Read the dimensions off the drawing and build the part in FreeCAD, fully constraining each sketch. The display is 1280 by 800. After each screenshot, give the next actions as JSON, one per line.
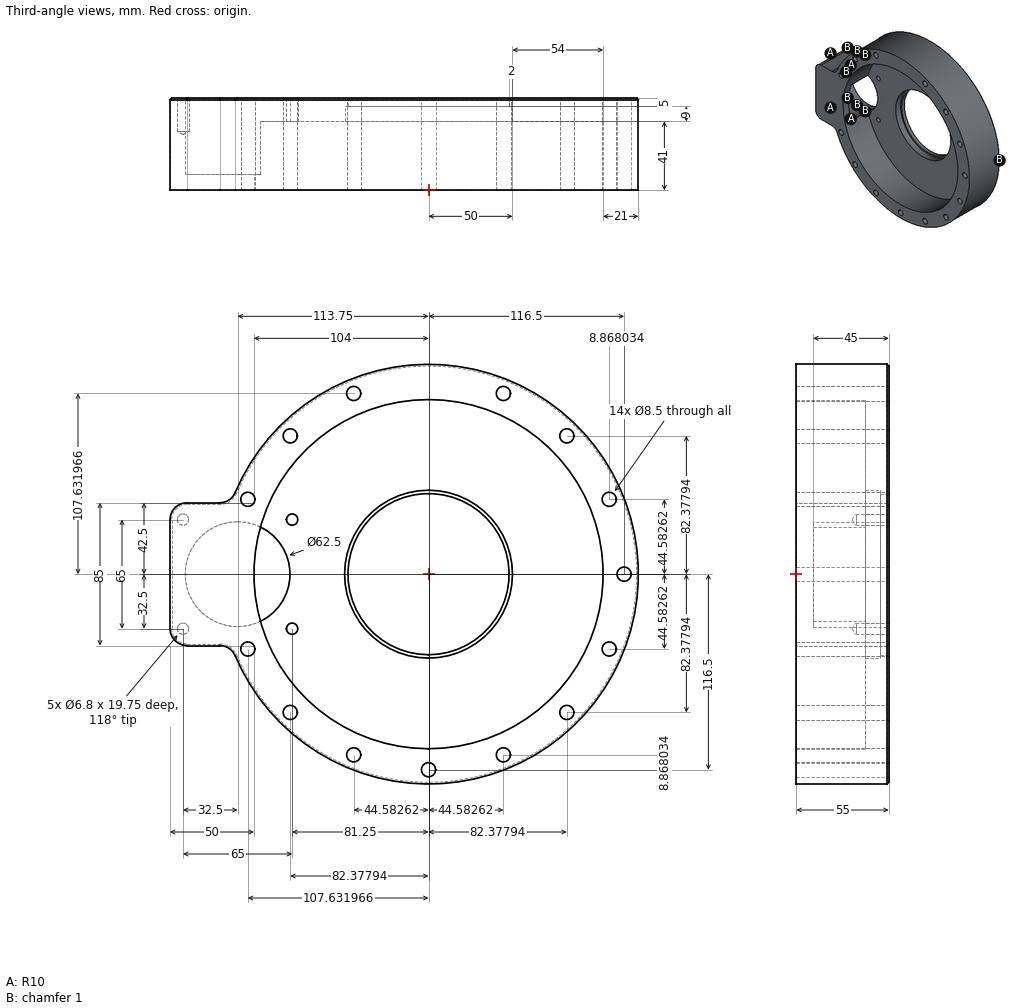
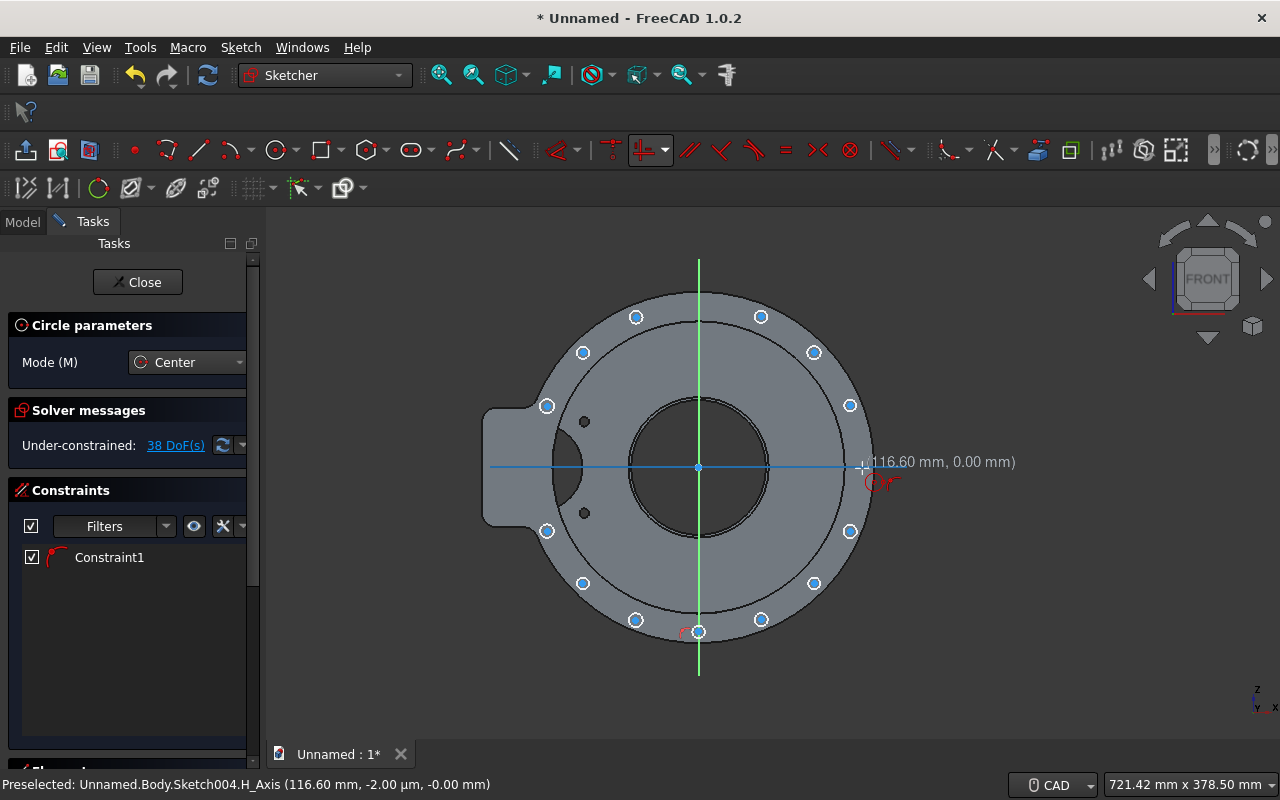
{"action": "left_click", "coordinate": [862, 467]}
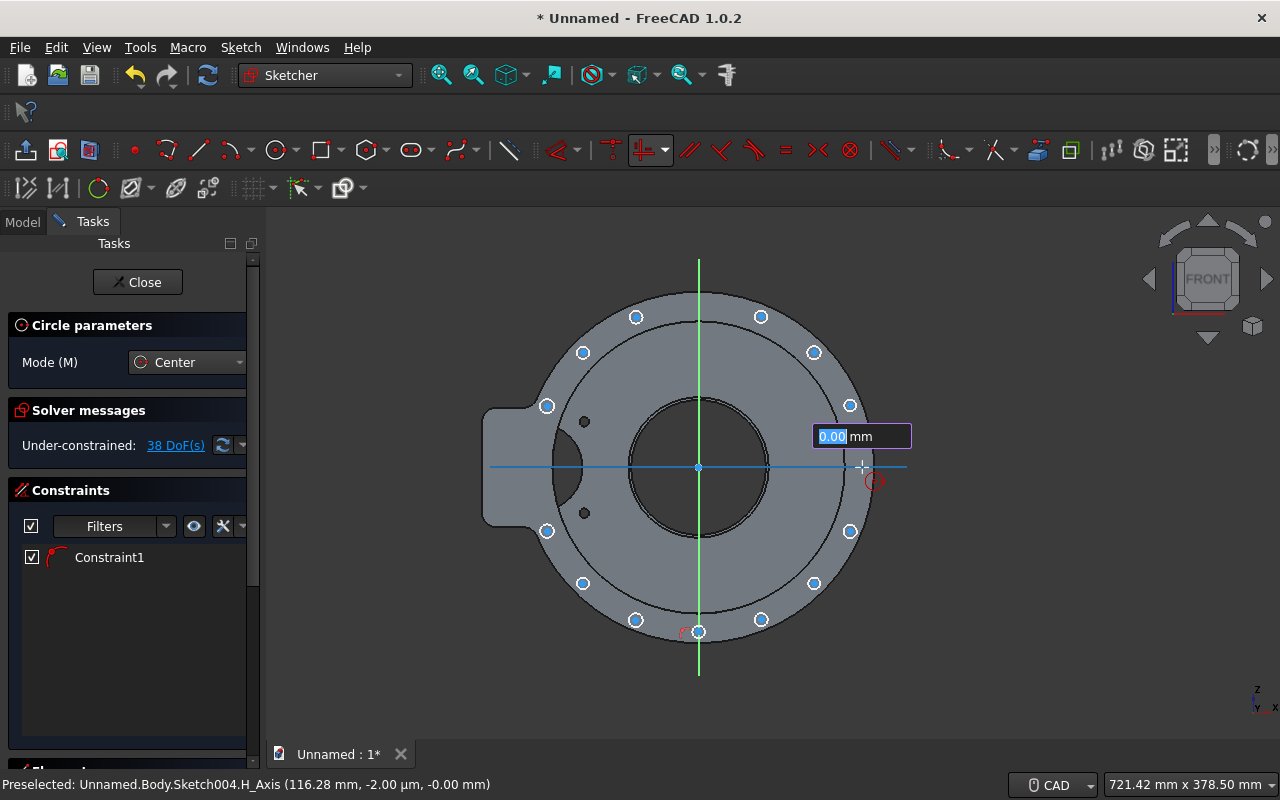
{"action": "scroll", "coordinate": [864, 462], "scroll_direction": "up", "scroll_amount": 6}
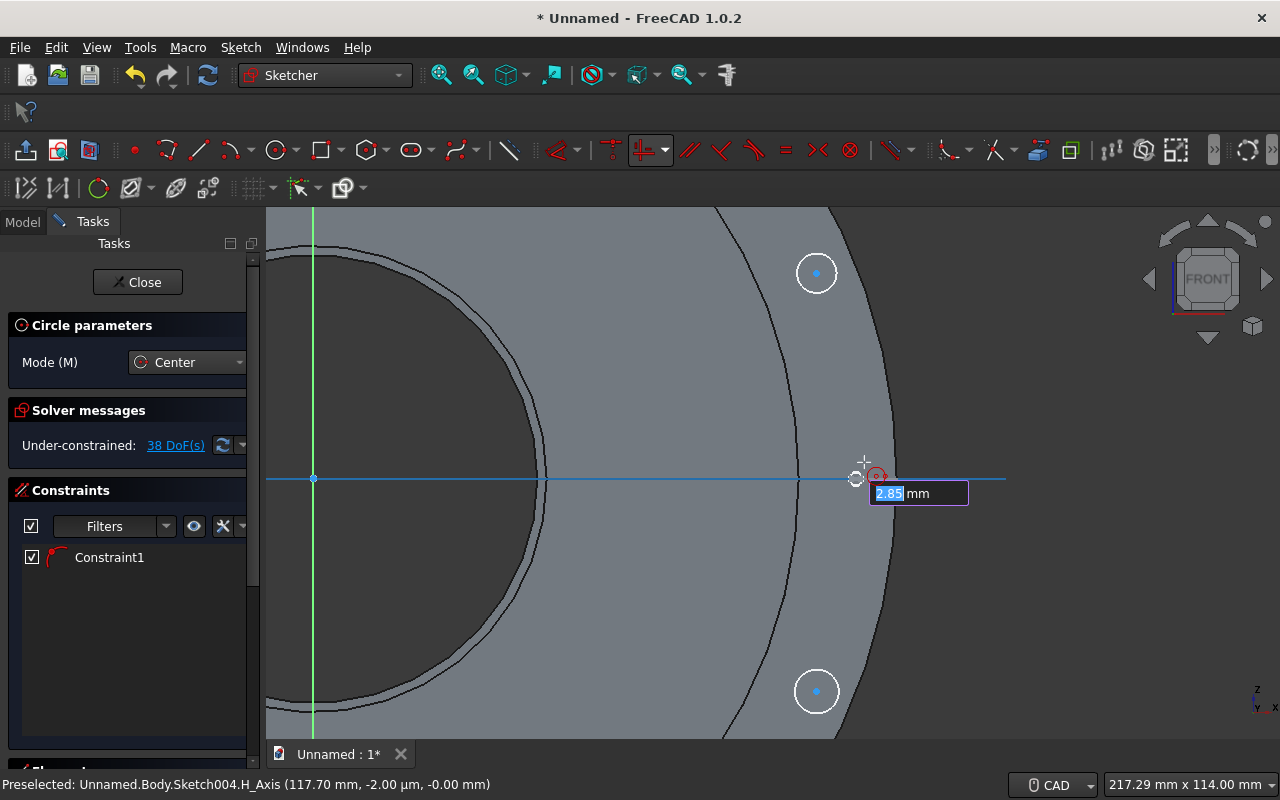
{"action": "left_click", "coordinate": [864, 460]}
{"action": "key", "text": "Escape"}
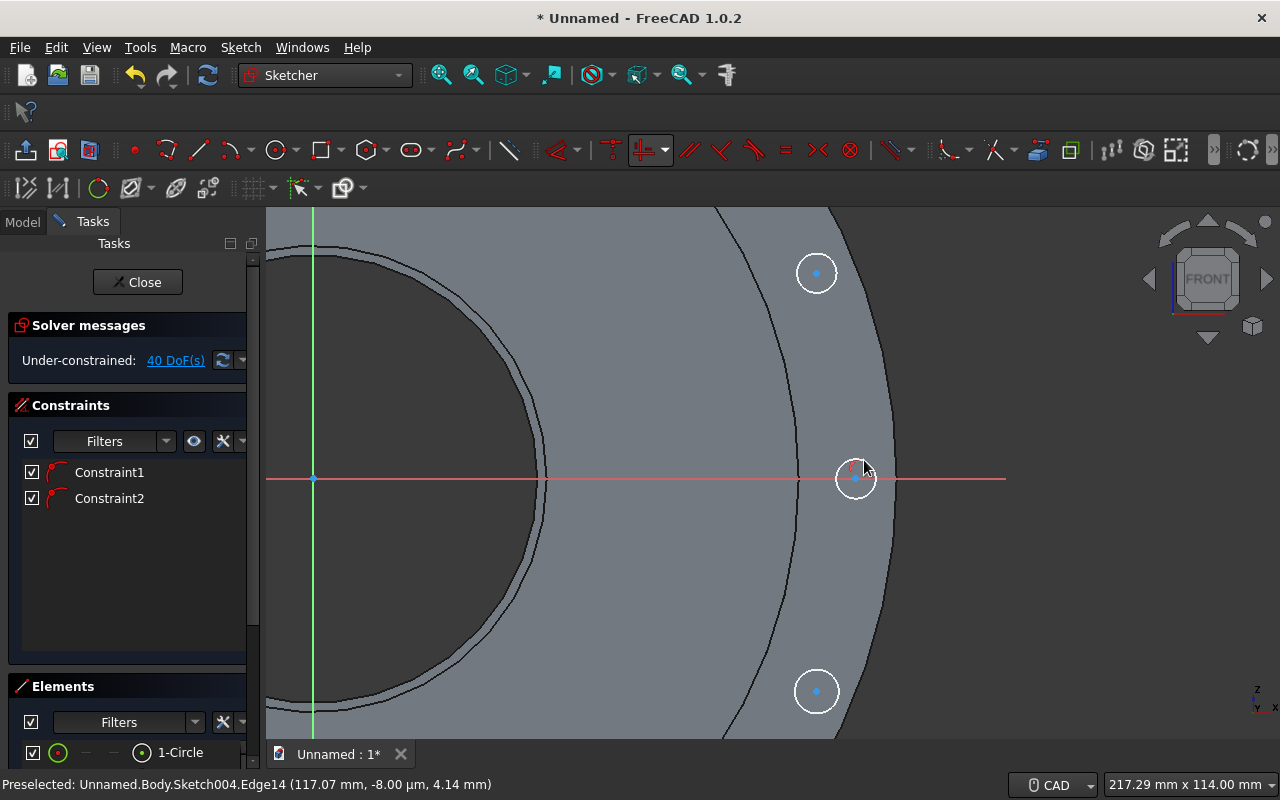
{"action": "left_click", "coordinate": [831, 259]}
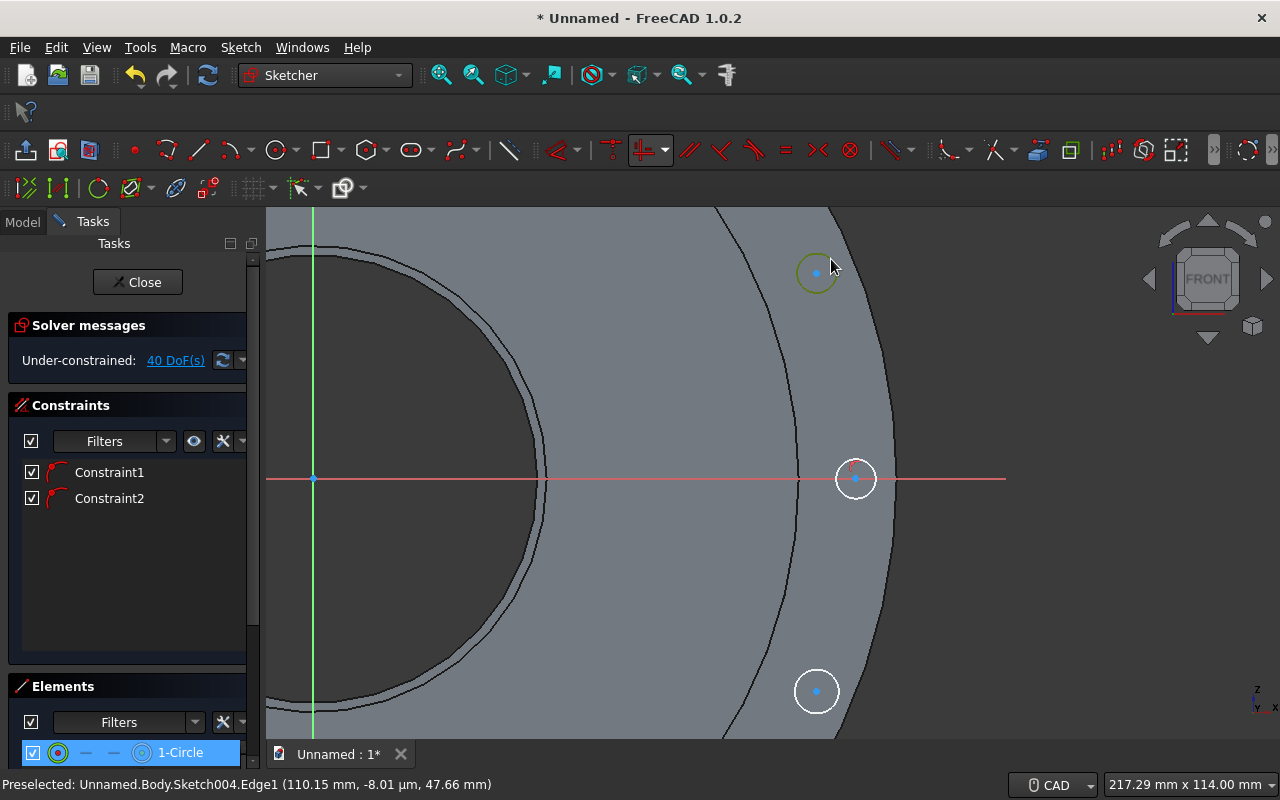
{"action": "left_click", "coordinate": [832, 676]}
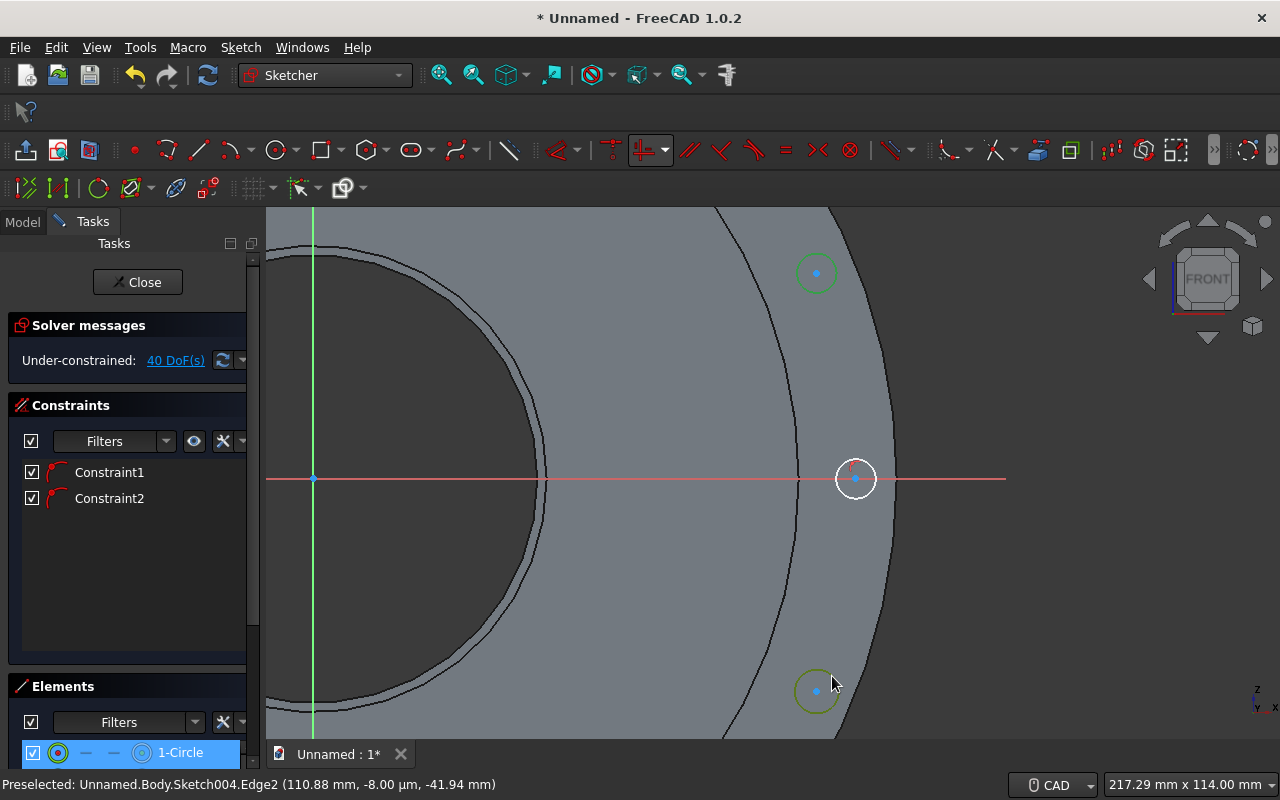
{"action": "scroll", "coordinate": [864, 462], "scroll_direction": "down", "scroll_amount": 6}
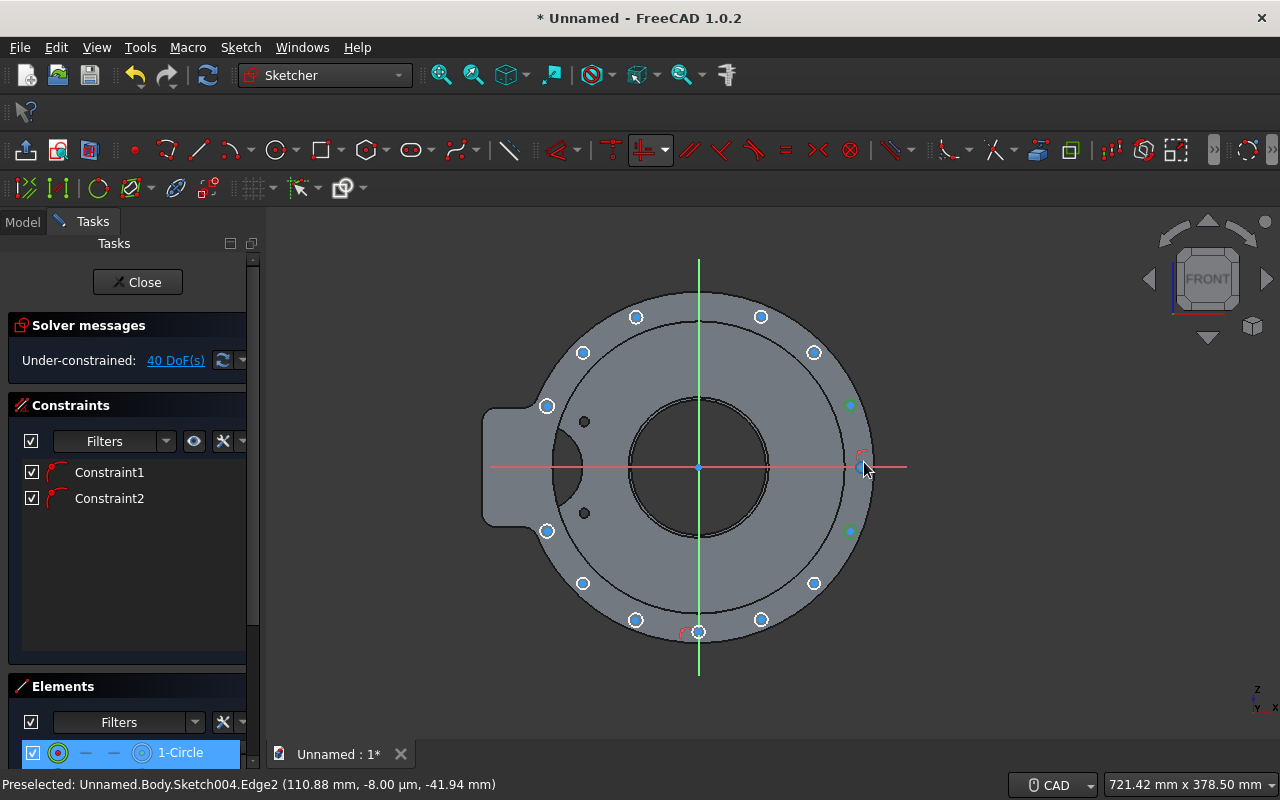
{"action": "scroll", "coordinate": [766, 615], "scroll_direction": "up", "scroll_amount": 4}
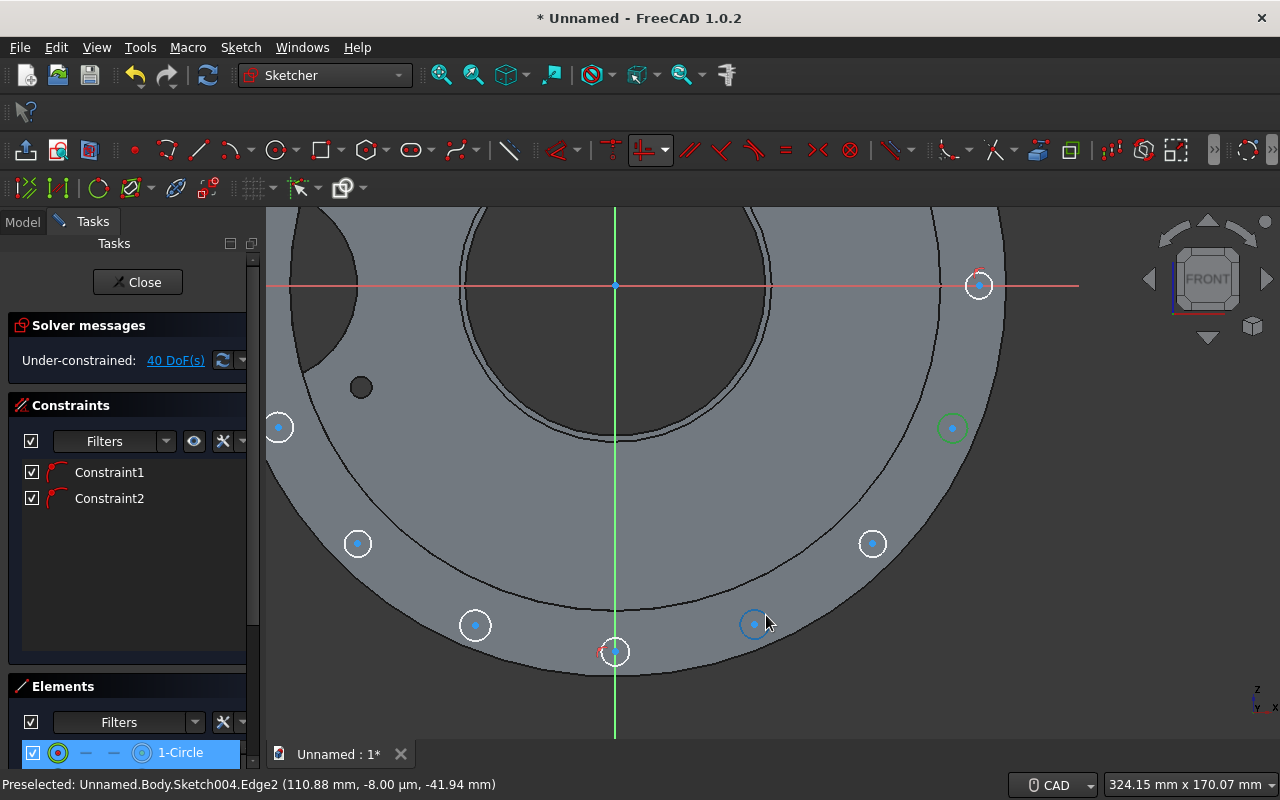
{"action": "left_click", "coordinate": [765, 614]}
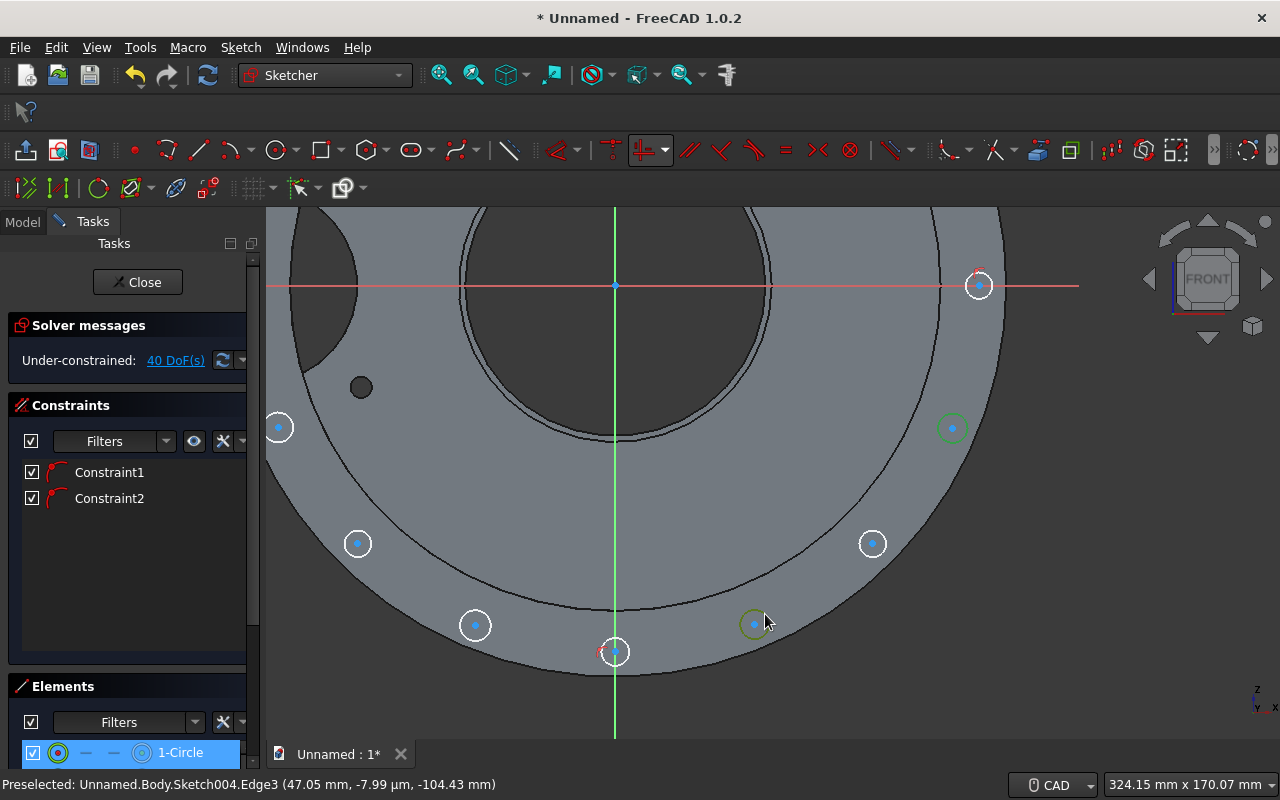
{"action": "left_click", "coordinate": [486, 615]}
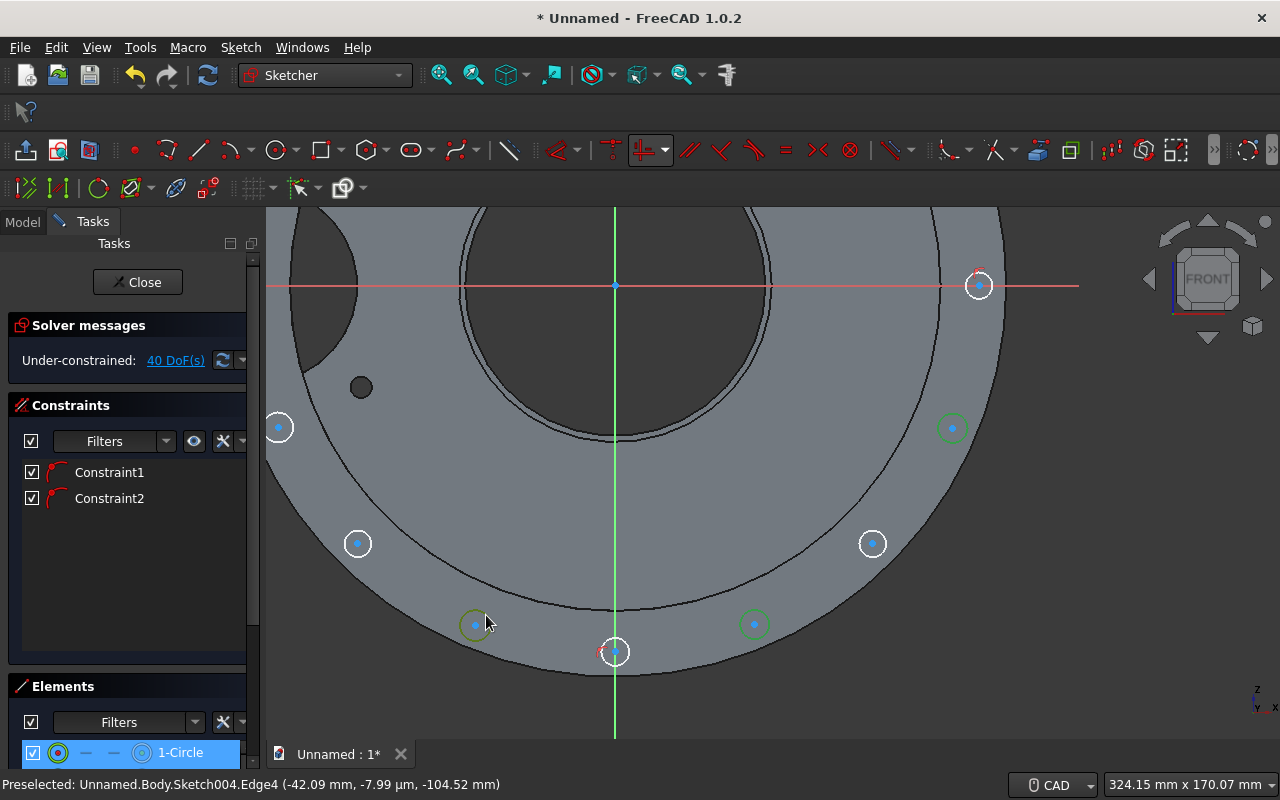
{"action": "scroll", "coordinate": [766, 615], "scroll_direction": "down", "scroll_amount": 4}